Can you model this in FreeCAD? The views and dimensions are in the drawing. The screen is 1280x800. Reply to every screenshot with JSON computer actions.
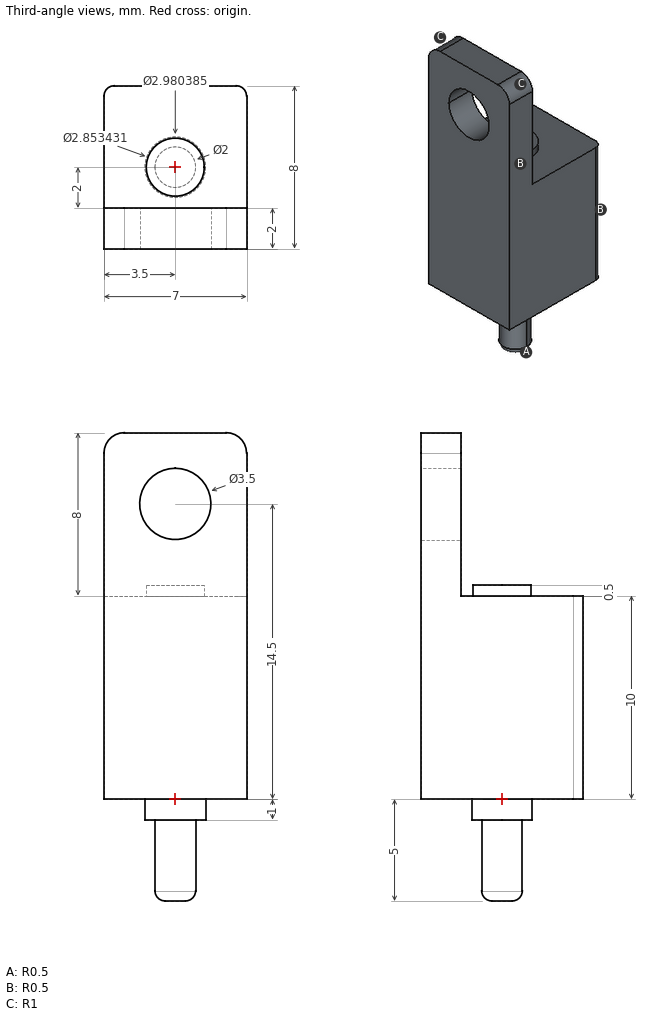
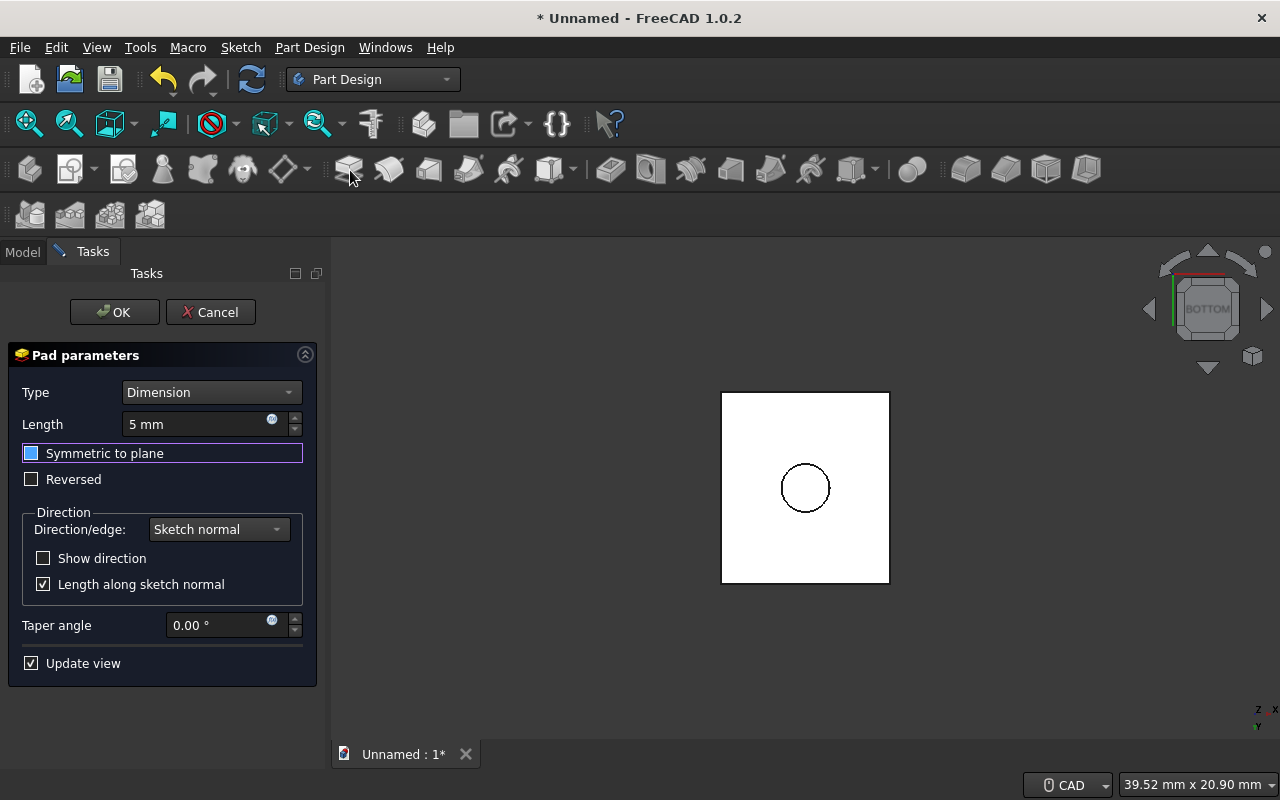
{"action": "left_click", "coordinate": [115, 312]}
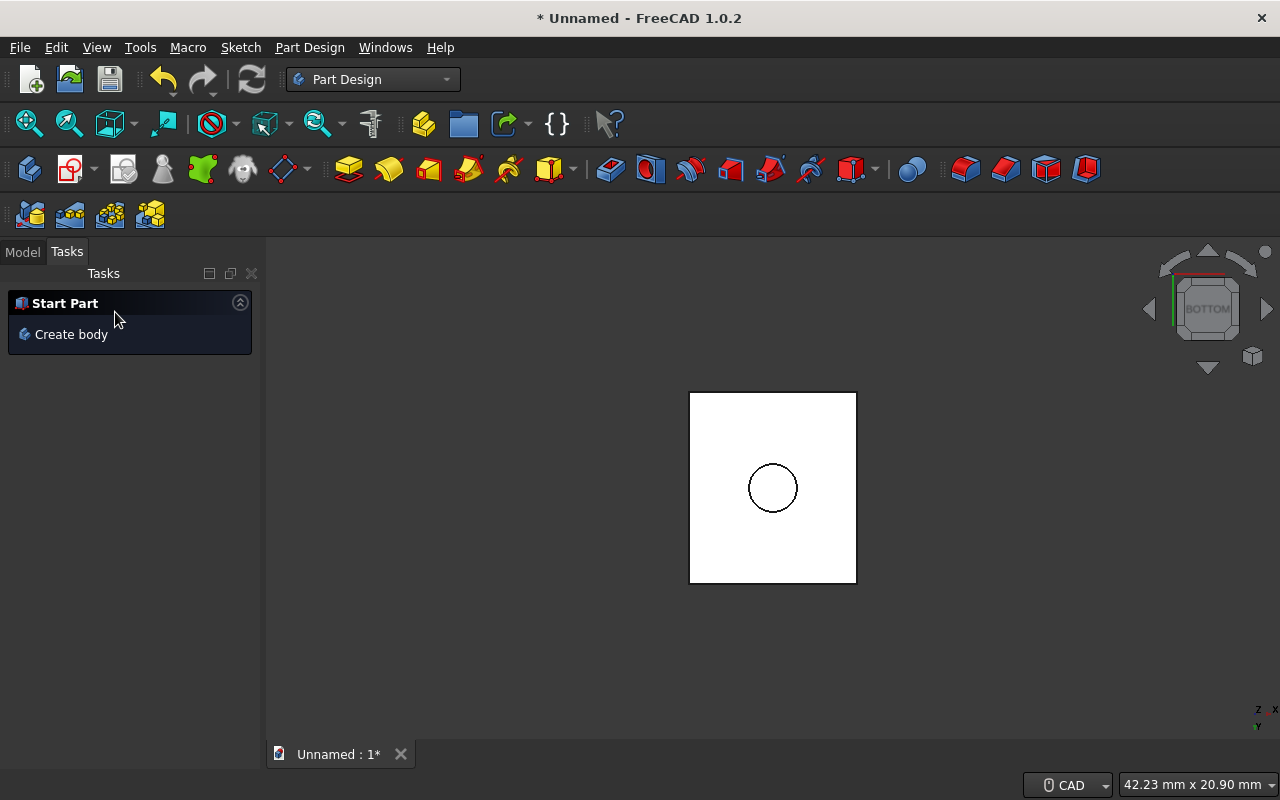
{"action": "key", "text": "v f"}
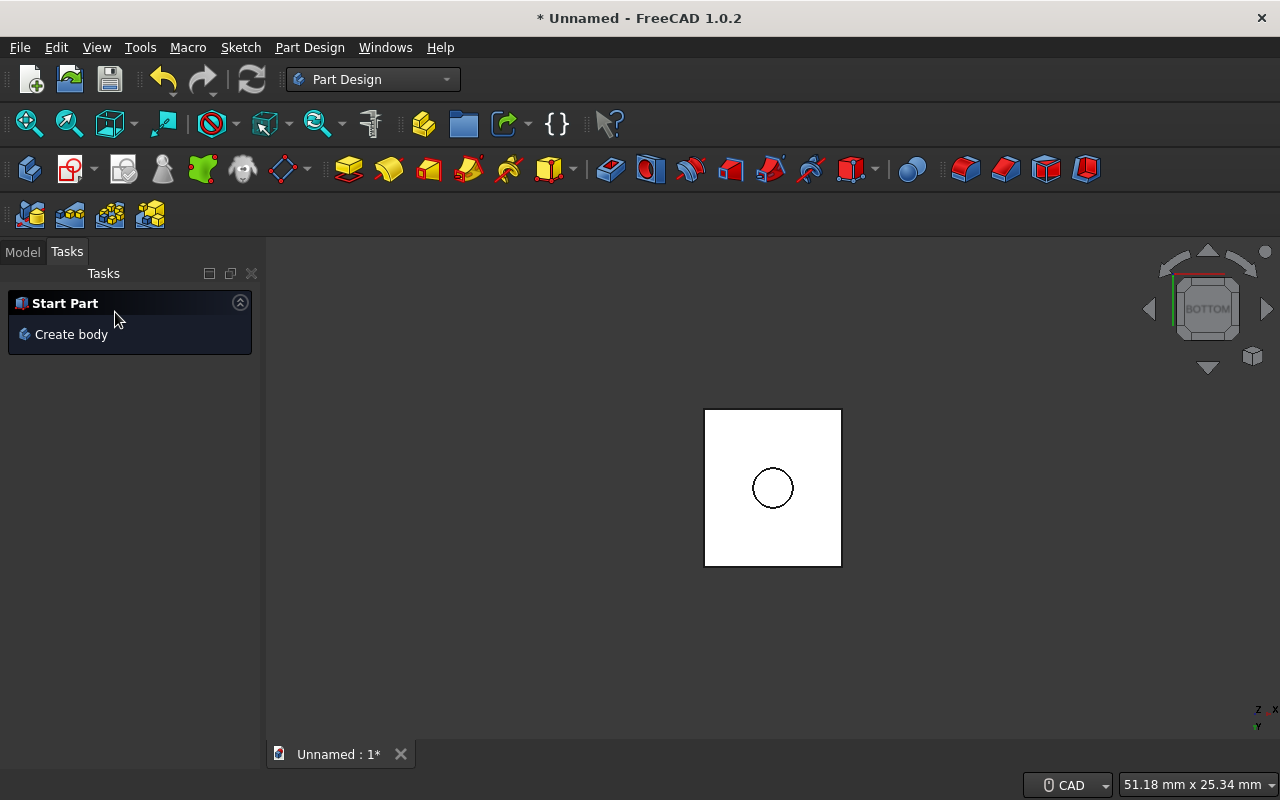
{"action": "left_click", "coordinate": [753, 487]}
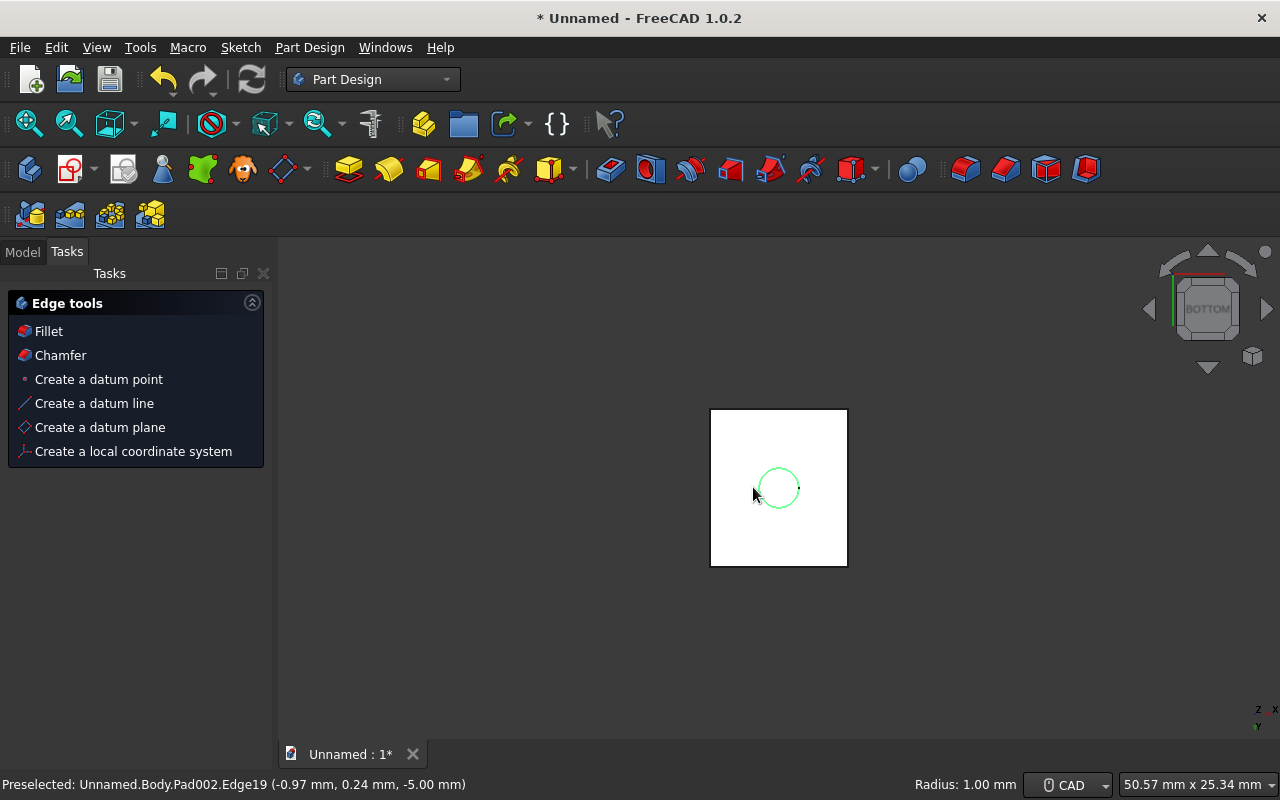
{"action": "left_click", "coordinate": [966, 170]}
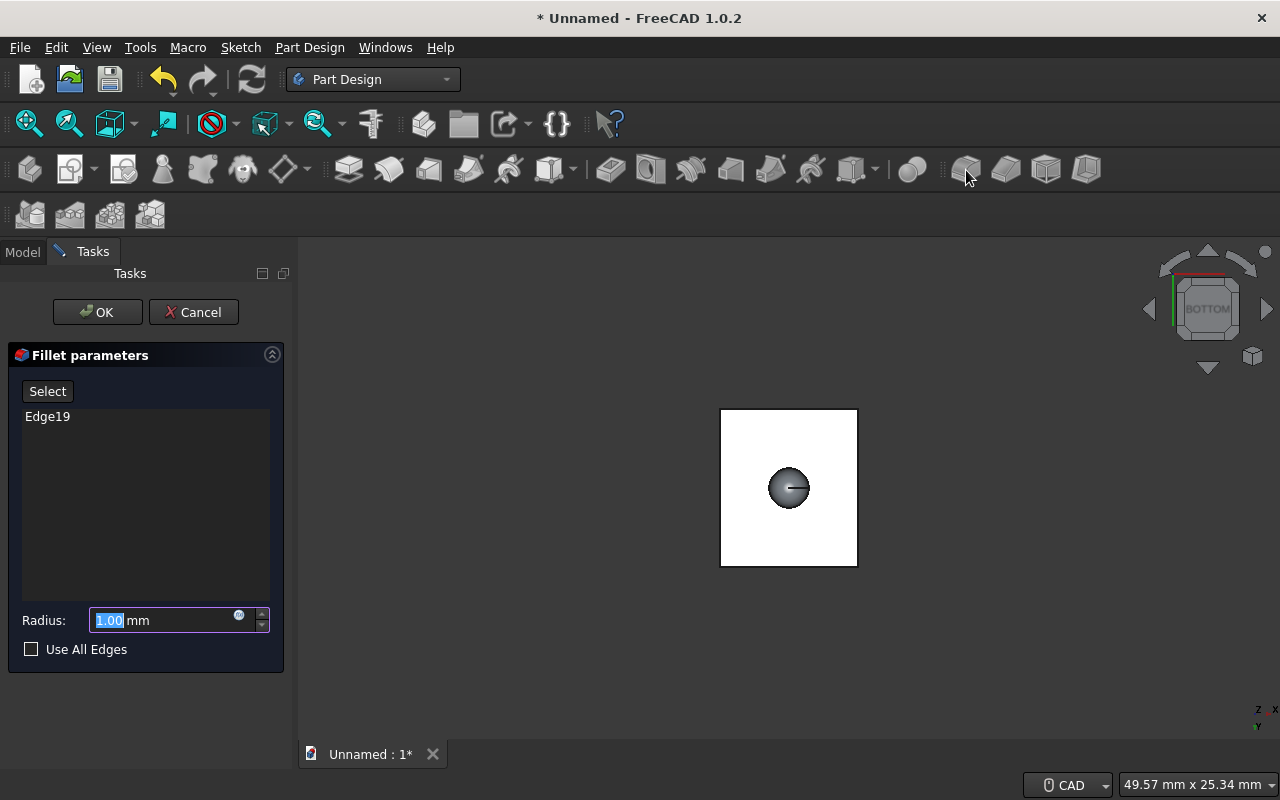
{"action": "type", "text": "0.5"}
{"action": "key", "text": "Tab"}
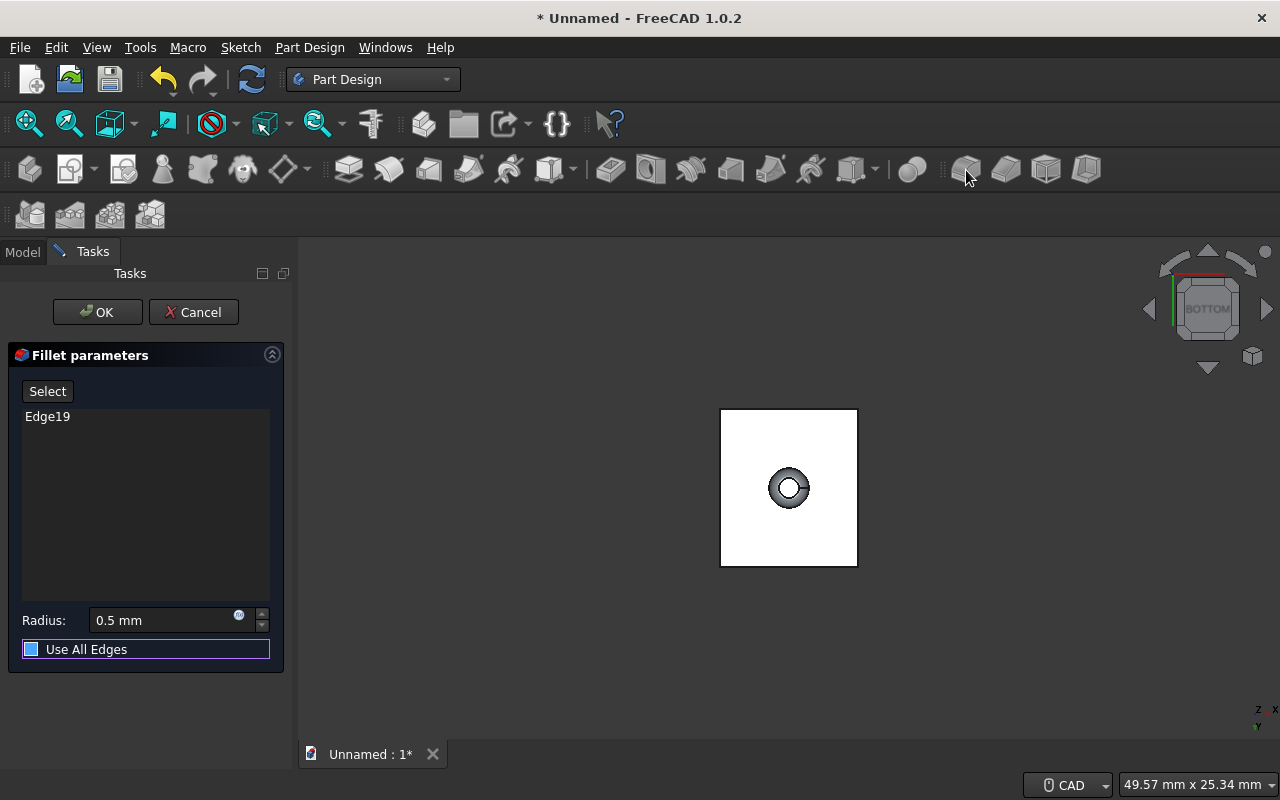
{"action": "left_click", "coordinate": [98, 312]}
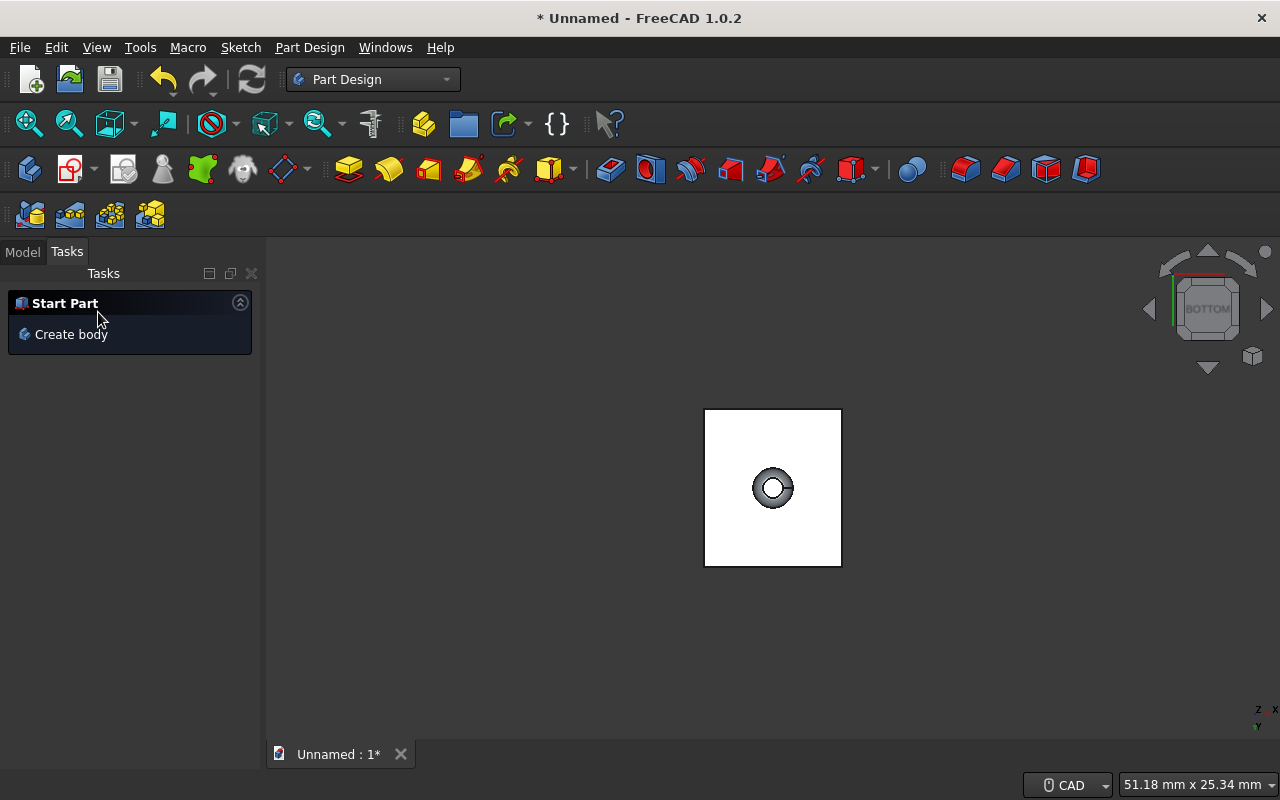
{"action": "key", "text": "v f"}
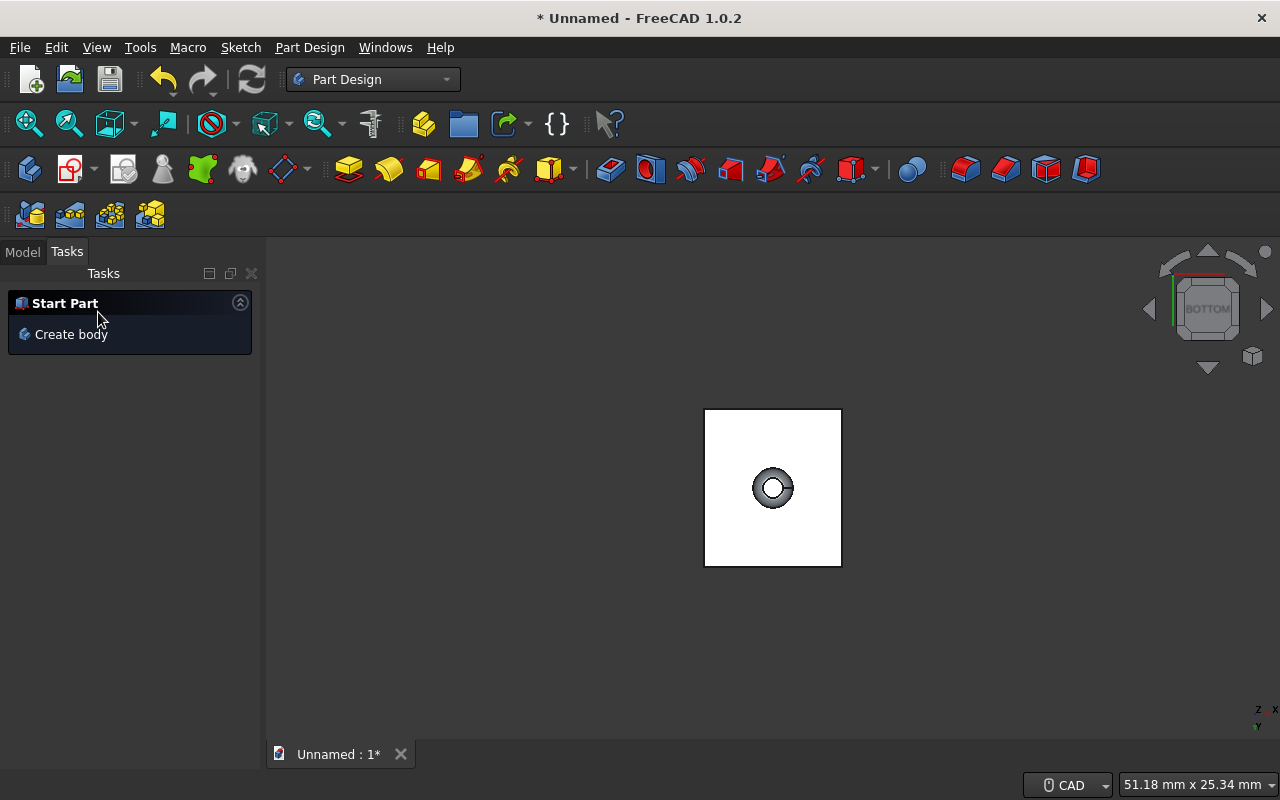
{"action": "left_click", "coordinate": [813, 532]}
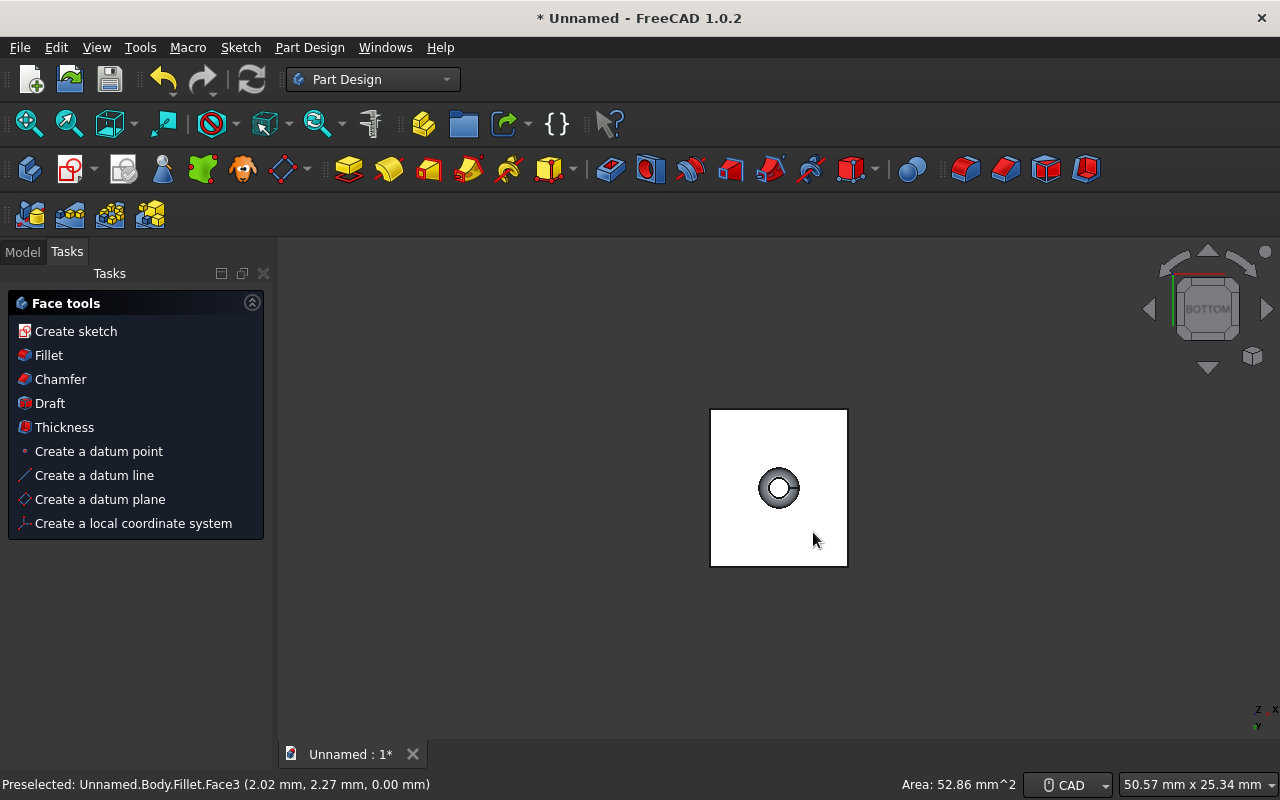
{"action": "left_click", "coordinate": [70, 170]}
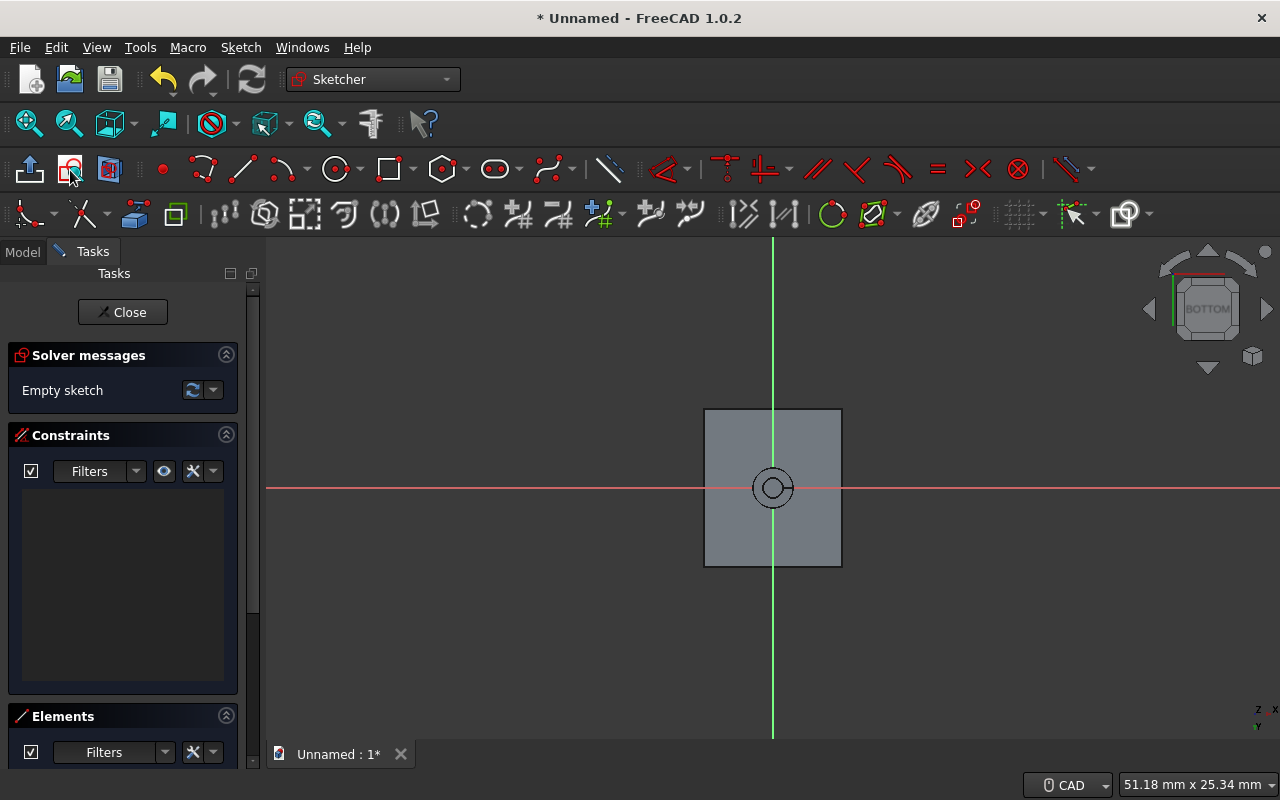
{"action": "key", "text": "q s"}